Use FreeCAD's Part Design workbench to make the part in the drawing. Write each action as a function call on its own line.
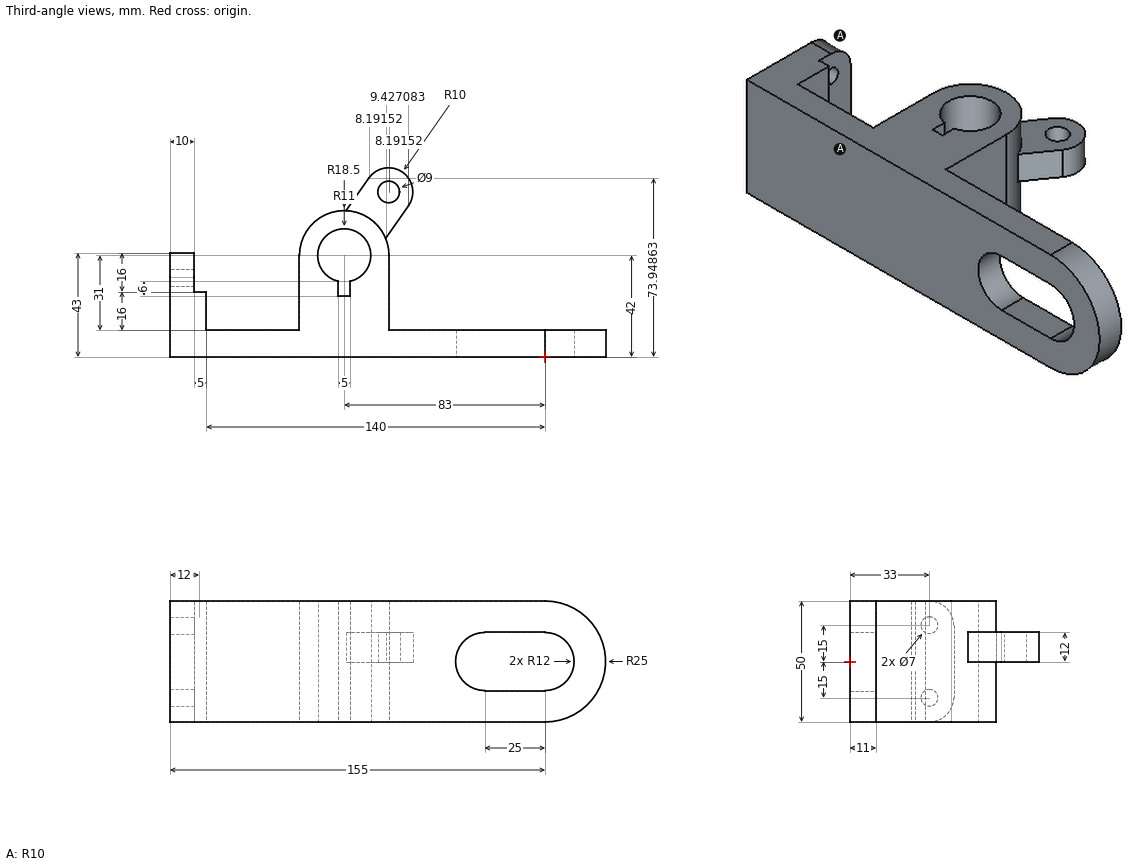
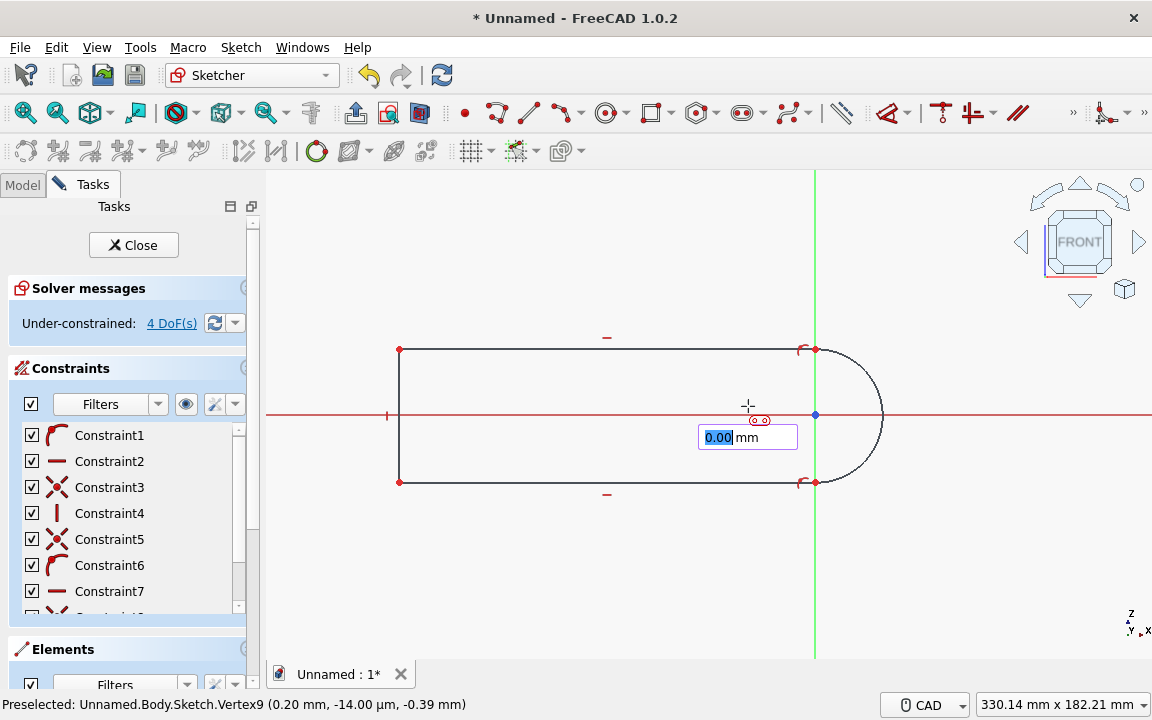
click(782, 383)
key(Escape)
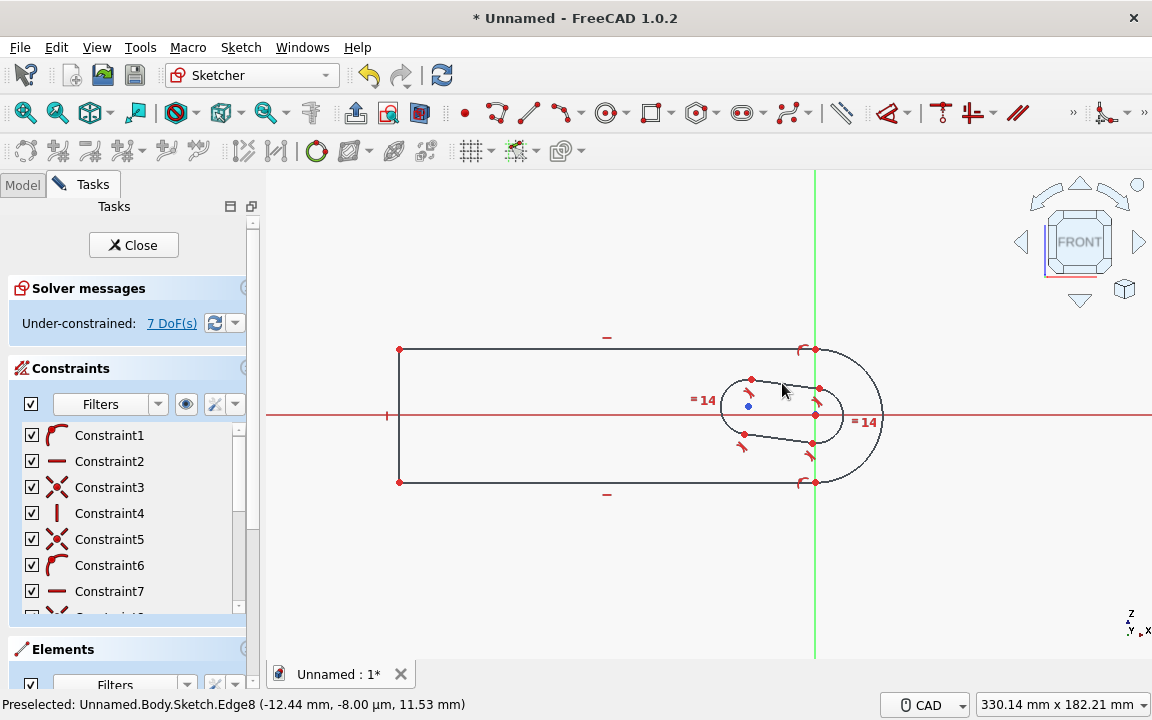
click(792, 440)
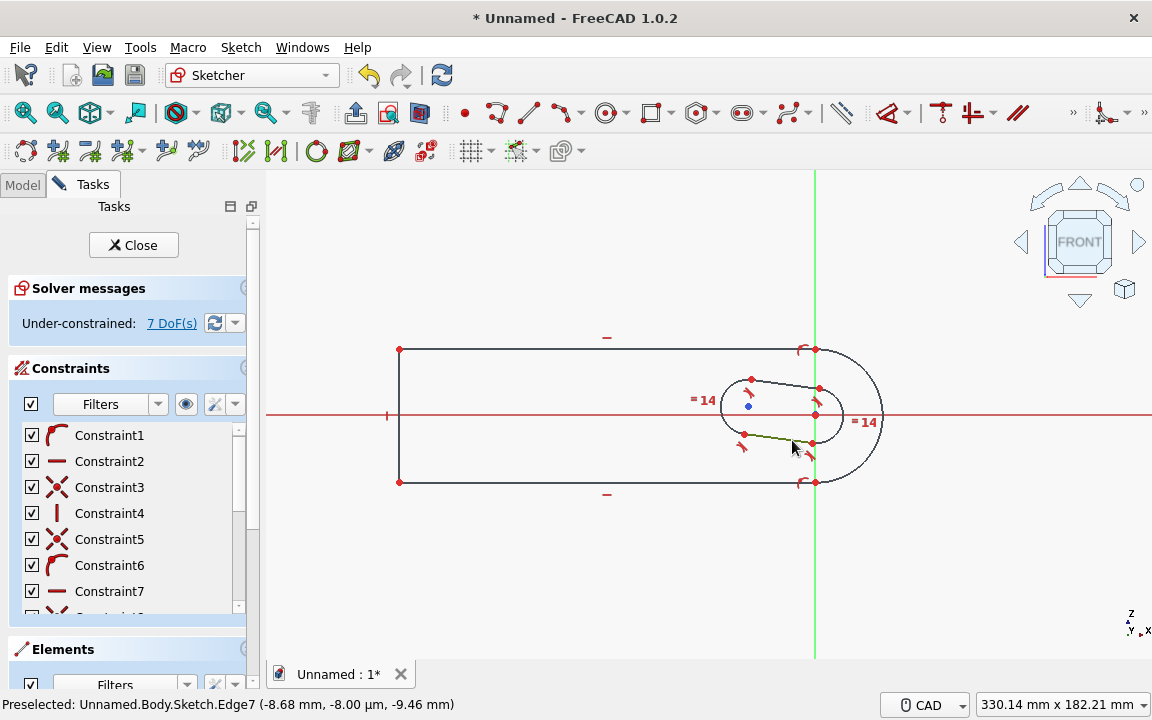
click(996, 114)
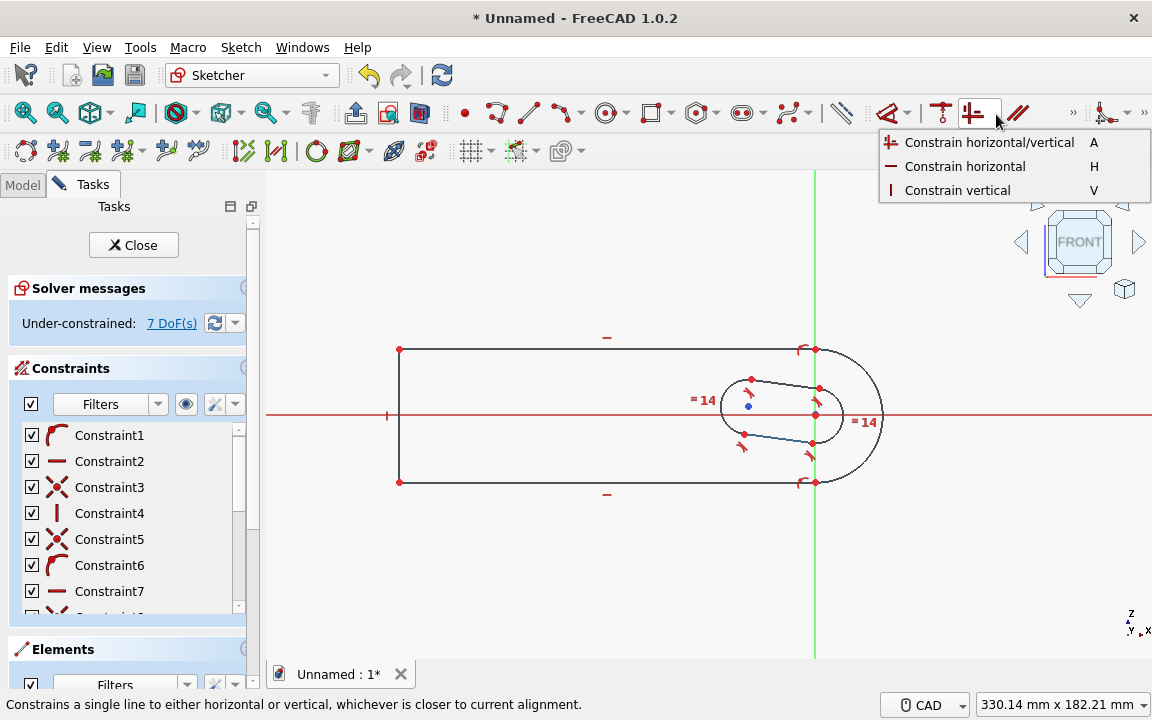
click(1015, 166)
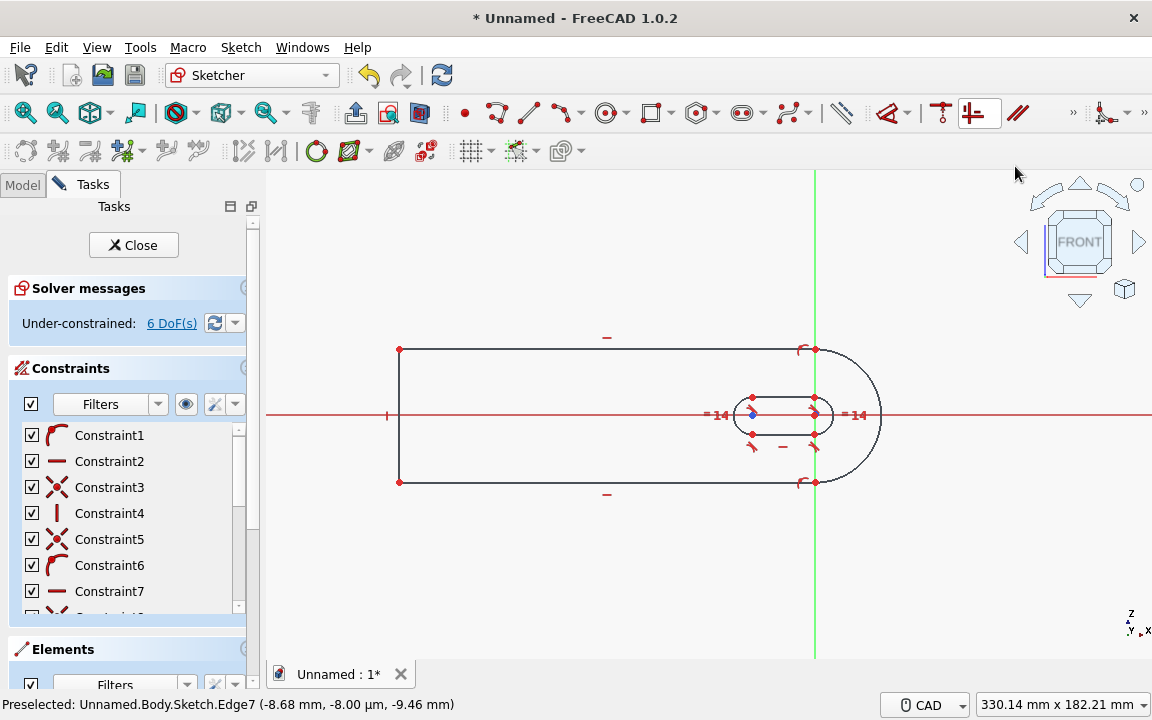
scroll(815, 415, up, 4)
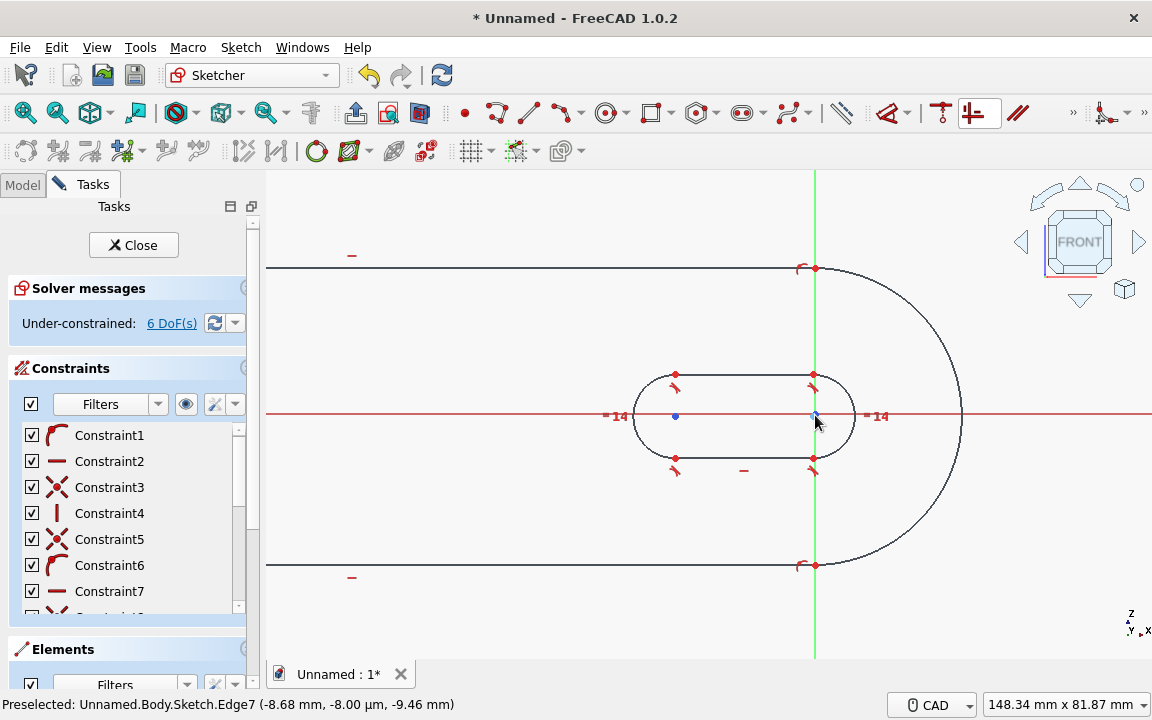
drag(803, 404, 825, 427)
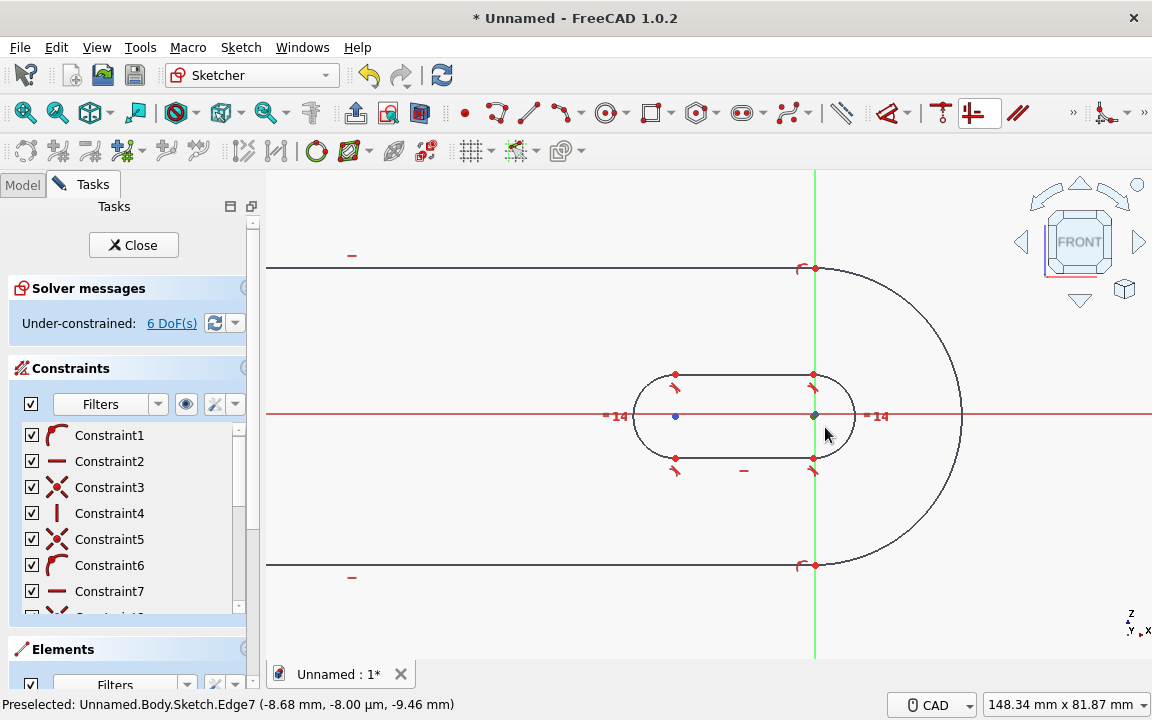
click(942, 114)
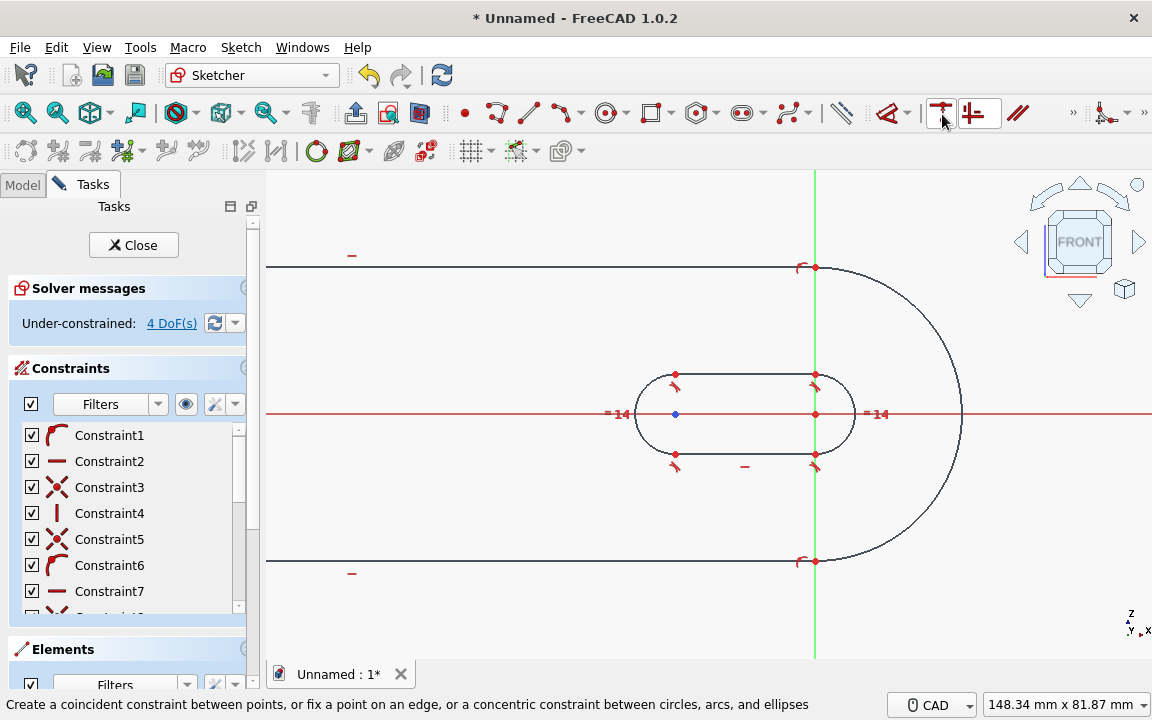
click(888, 114)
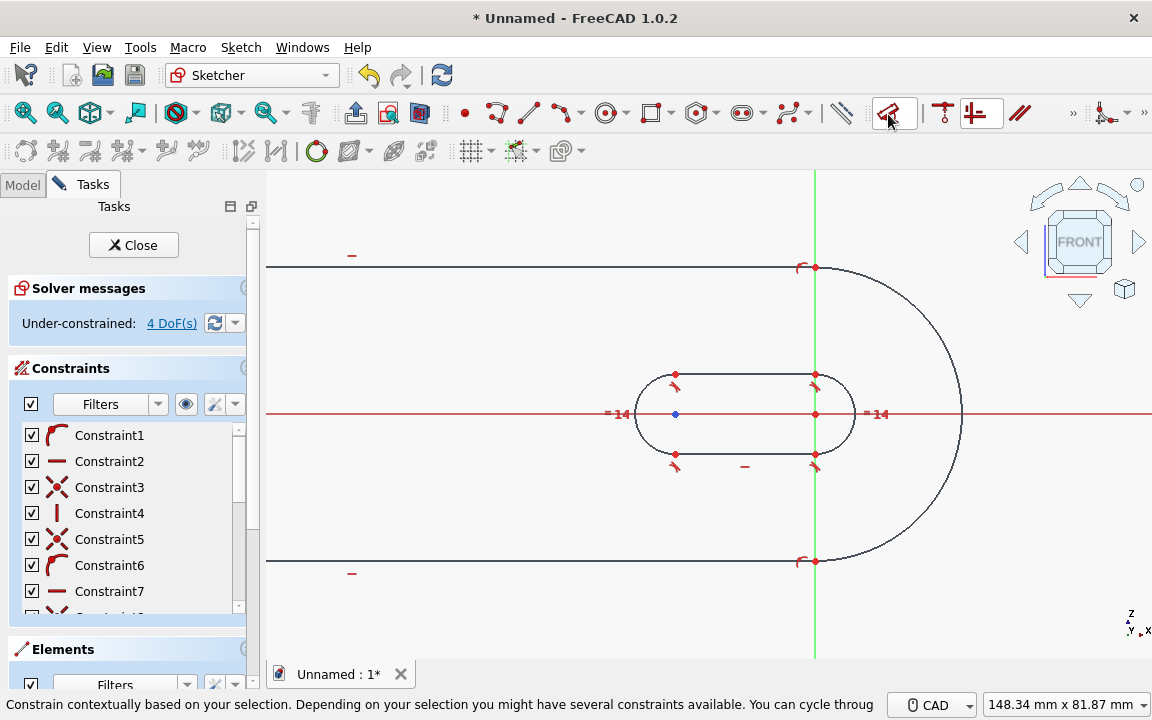
click(934, 501)
click(960, 520)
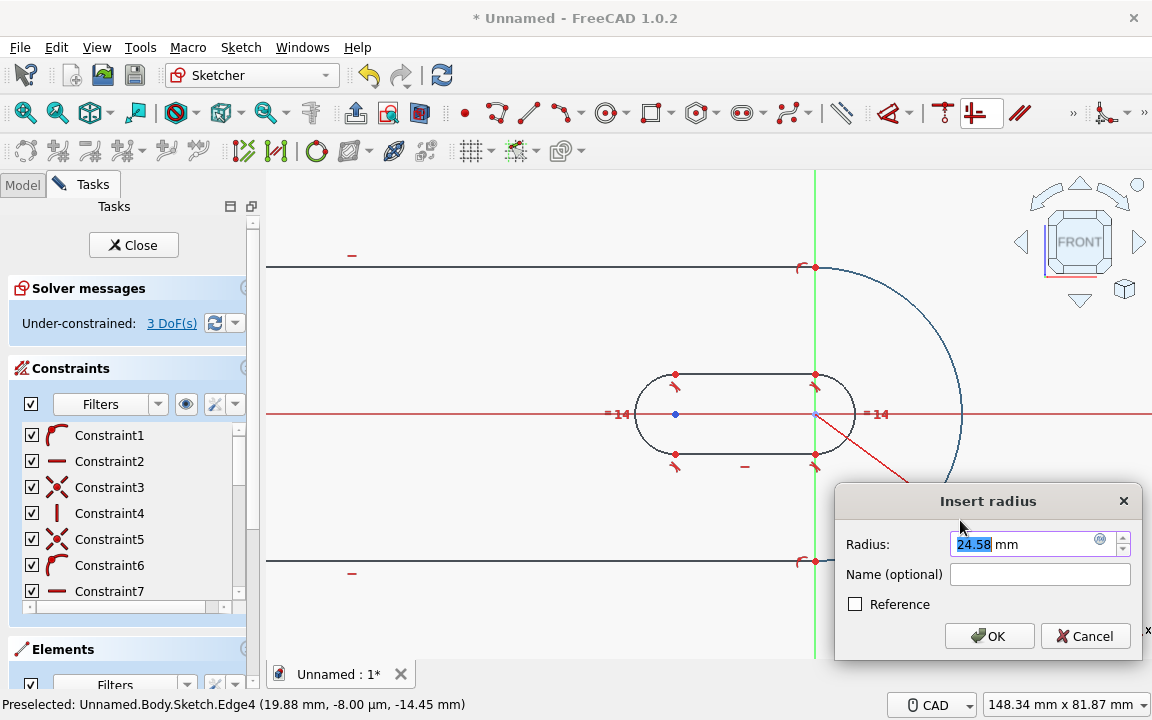
text(25)
key(Return)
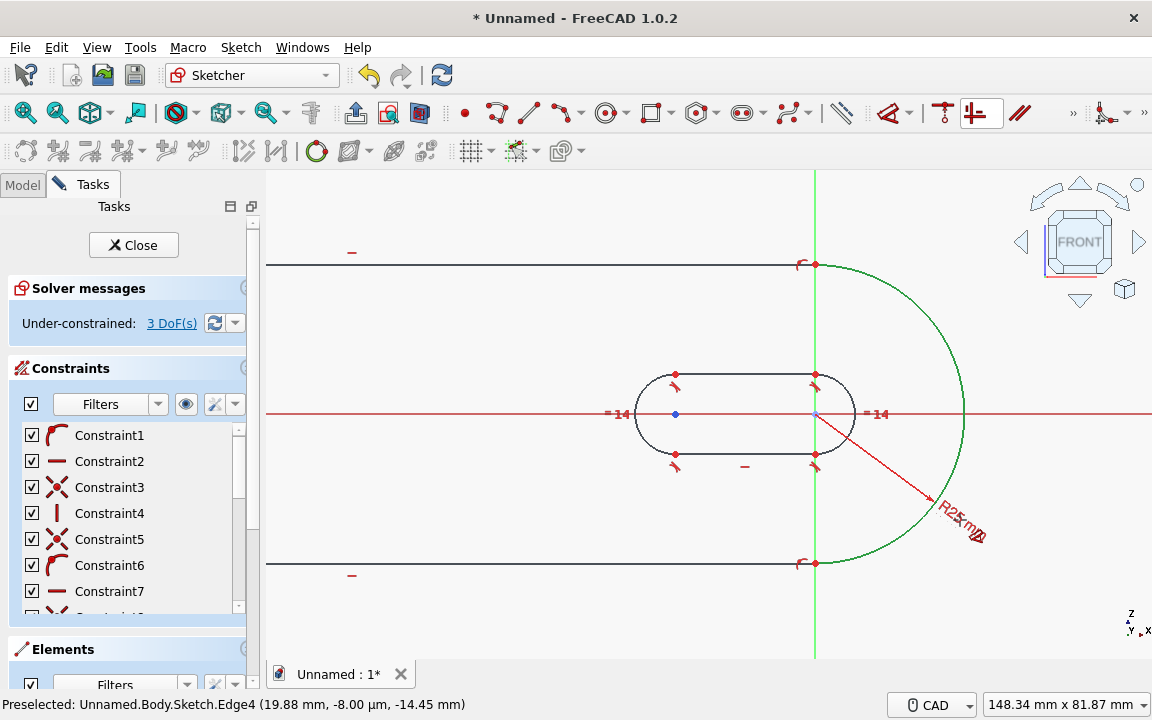
click(847, 438)
click(873, 457)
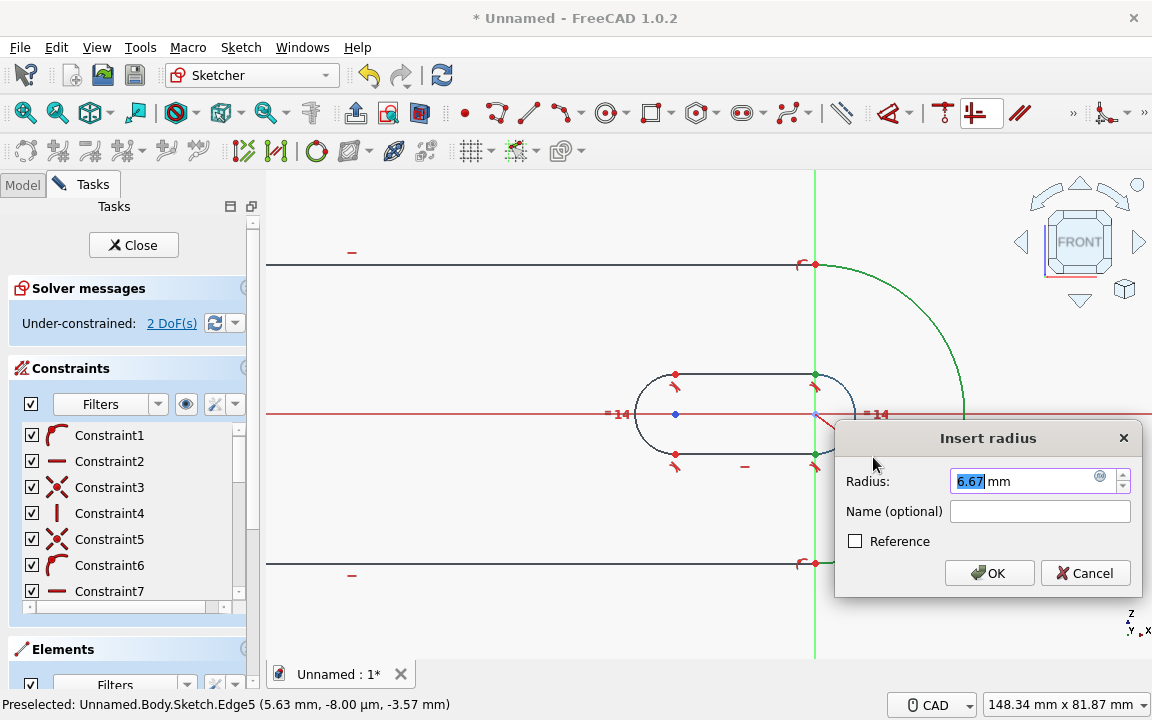
text(12)
key(Return)